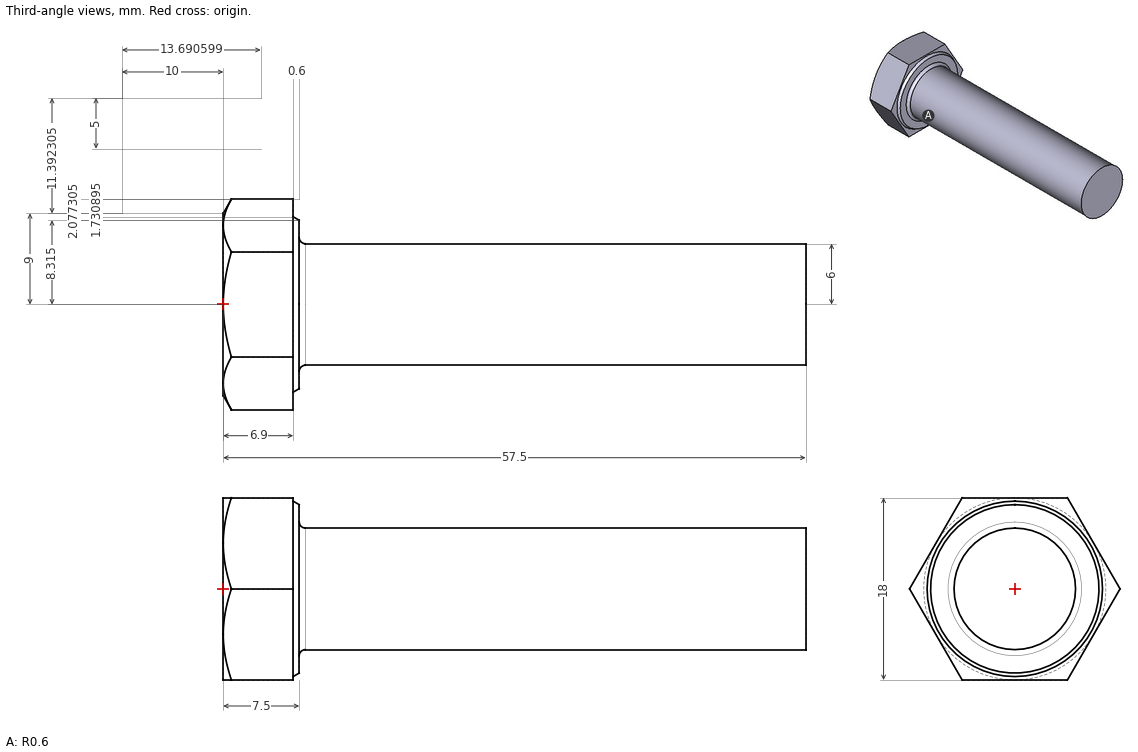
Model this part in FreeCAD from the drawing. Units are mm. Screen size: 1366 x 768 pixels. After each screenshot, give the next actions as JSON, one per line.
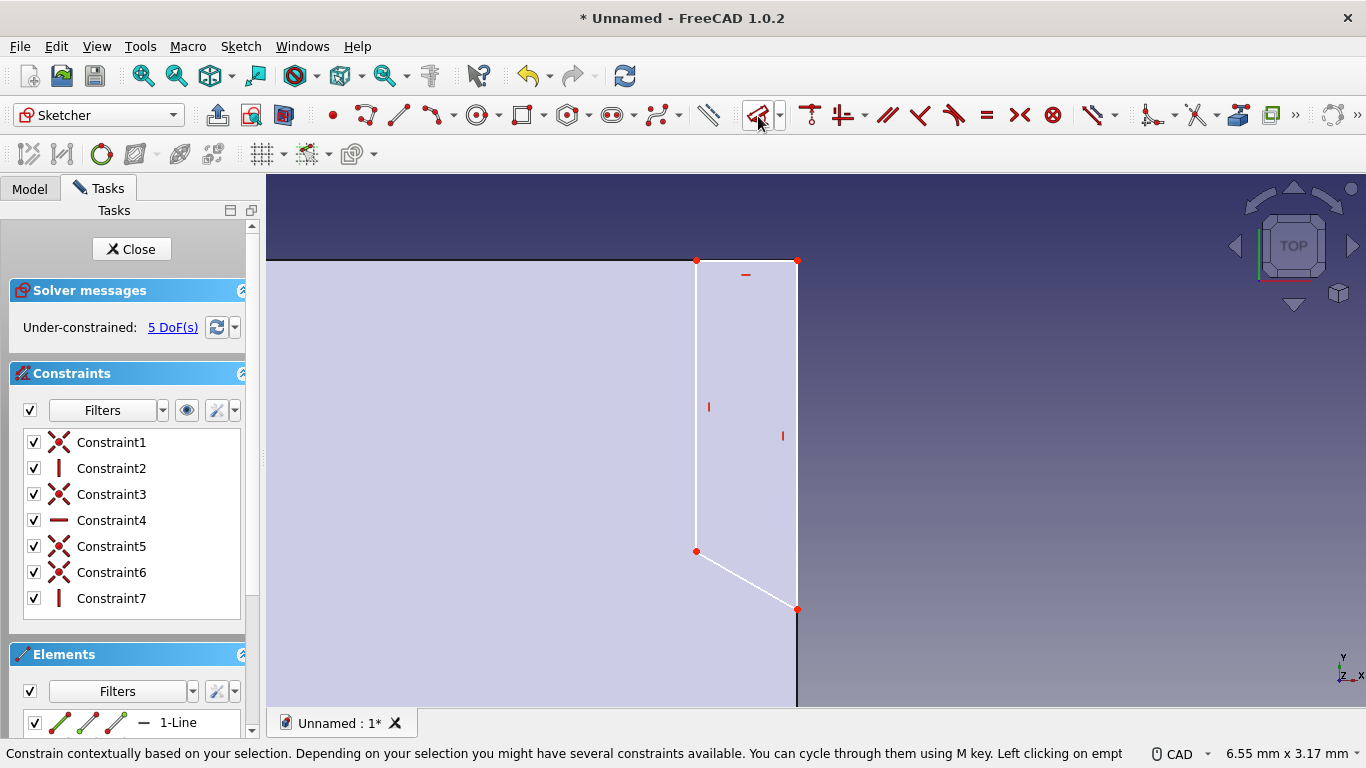
{"action": "left_click", "coordinate": [767, 261]}
{"action": "left_click", "coordinate": [746, 227]}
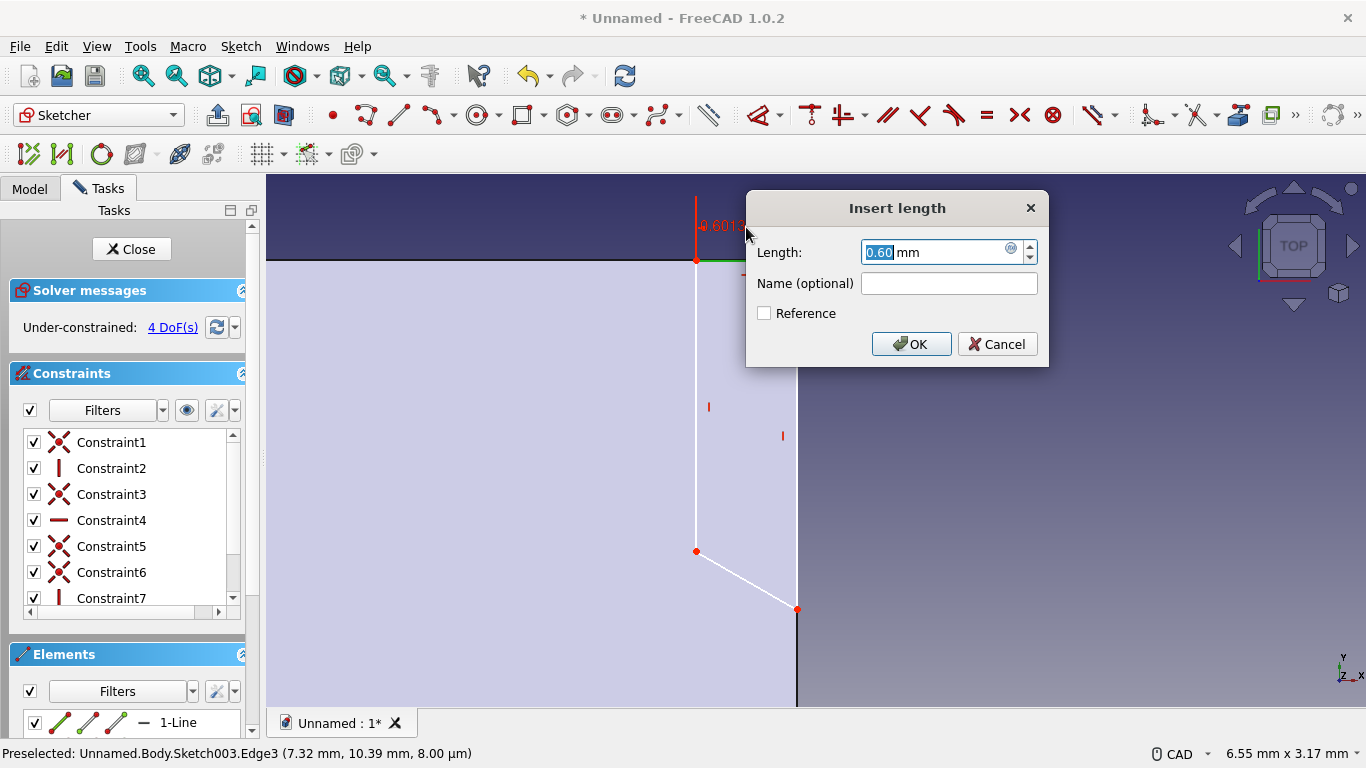
{"action": "type", "text": "0.6"}
{"action": "key", "text": "Return"}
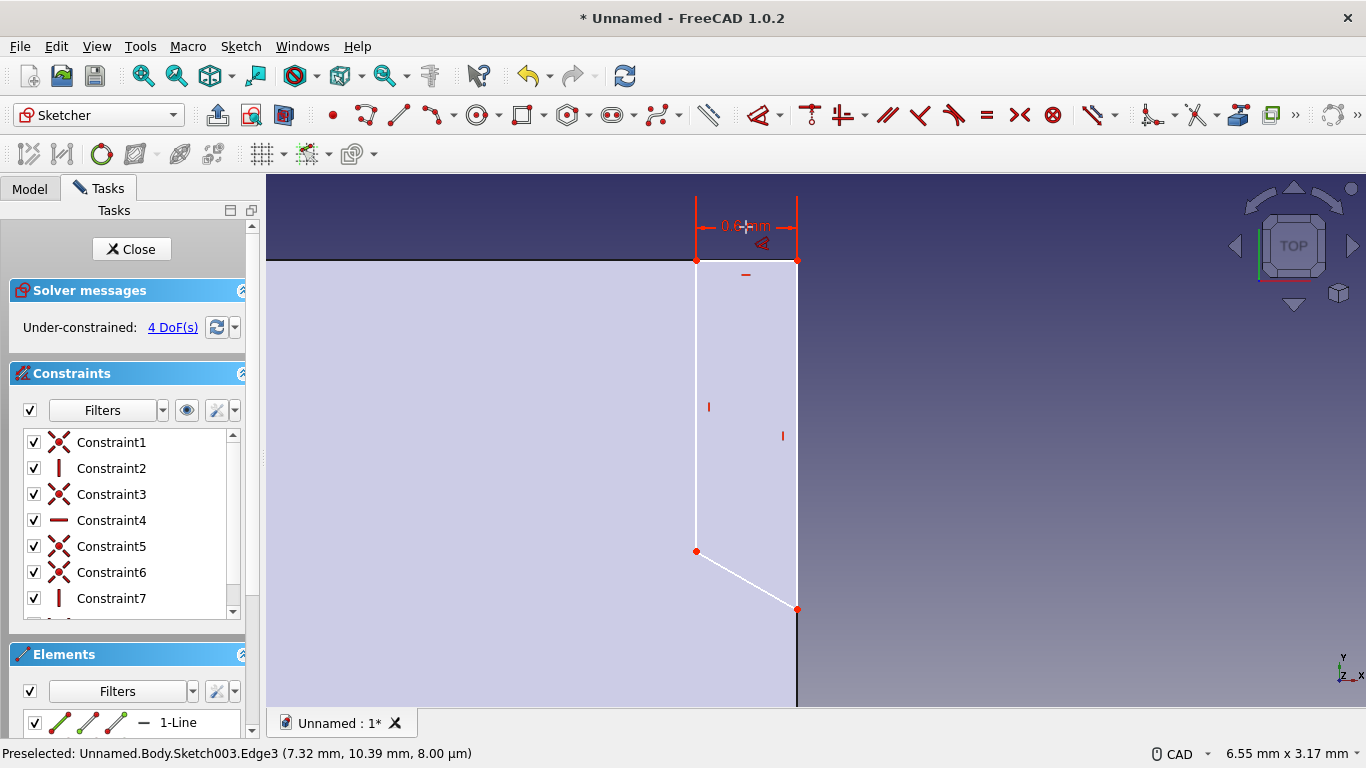
{"action": "left_click", "coordinate": [696, 552]}
{"action": "left_click", "coordinate": [495, 518]}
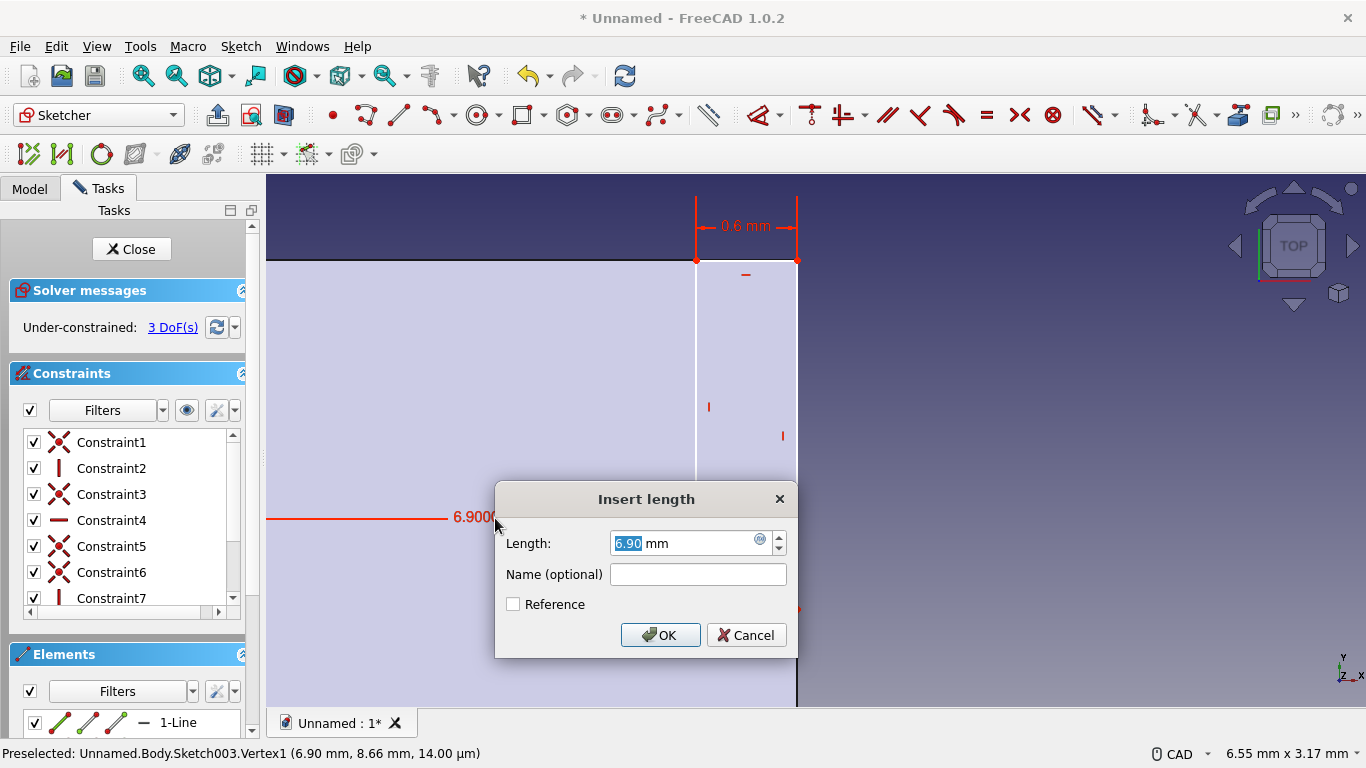
{"action": "type", "text": "6.9"}
{"action": "key", "text": "Return"}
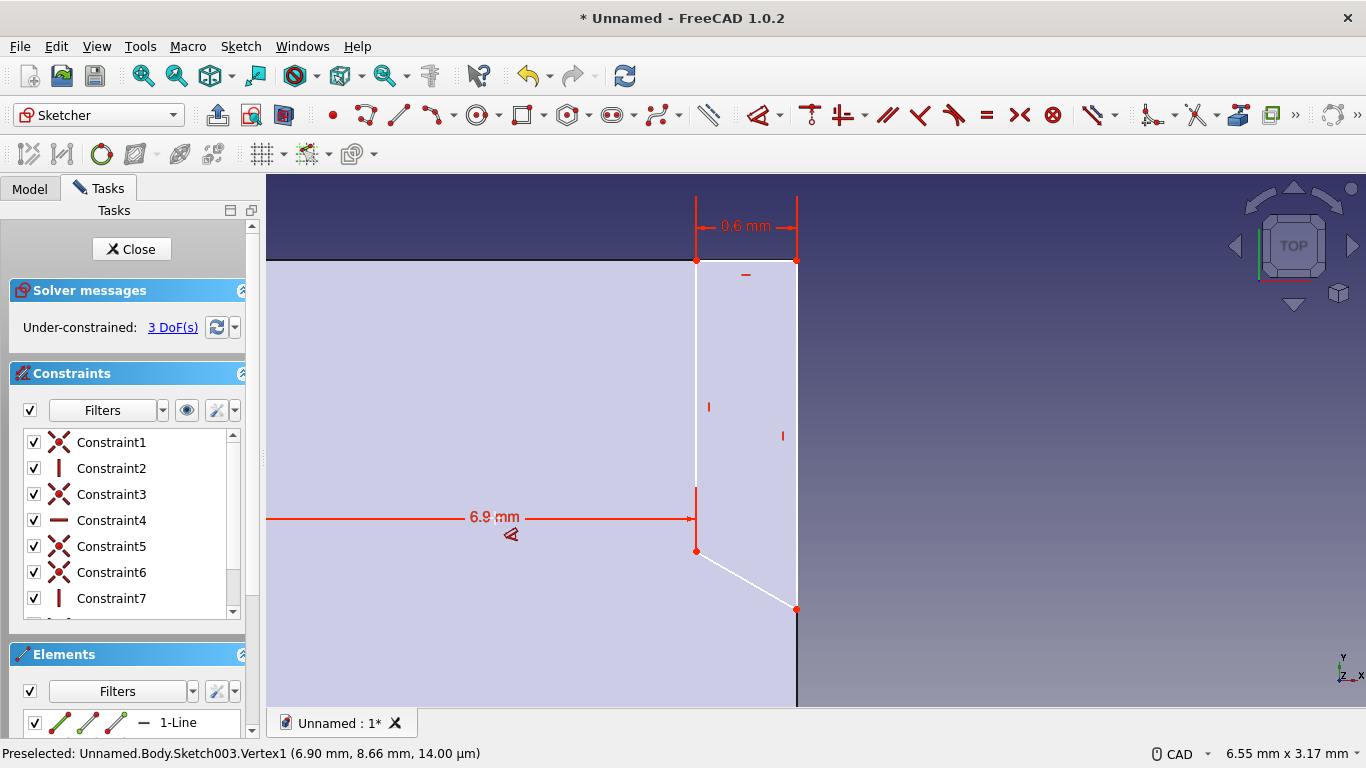
{"action": "left_click", "coordinate": [797, 610]}
{"action": "left_click", "coordinate": [831, 644]}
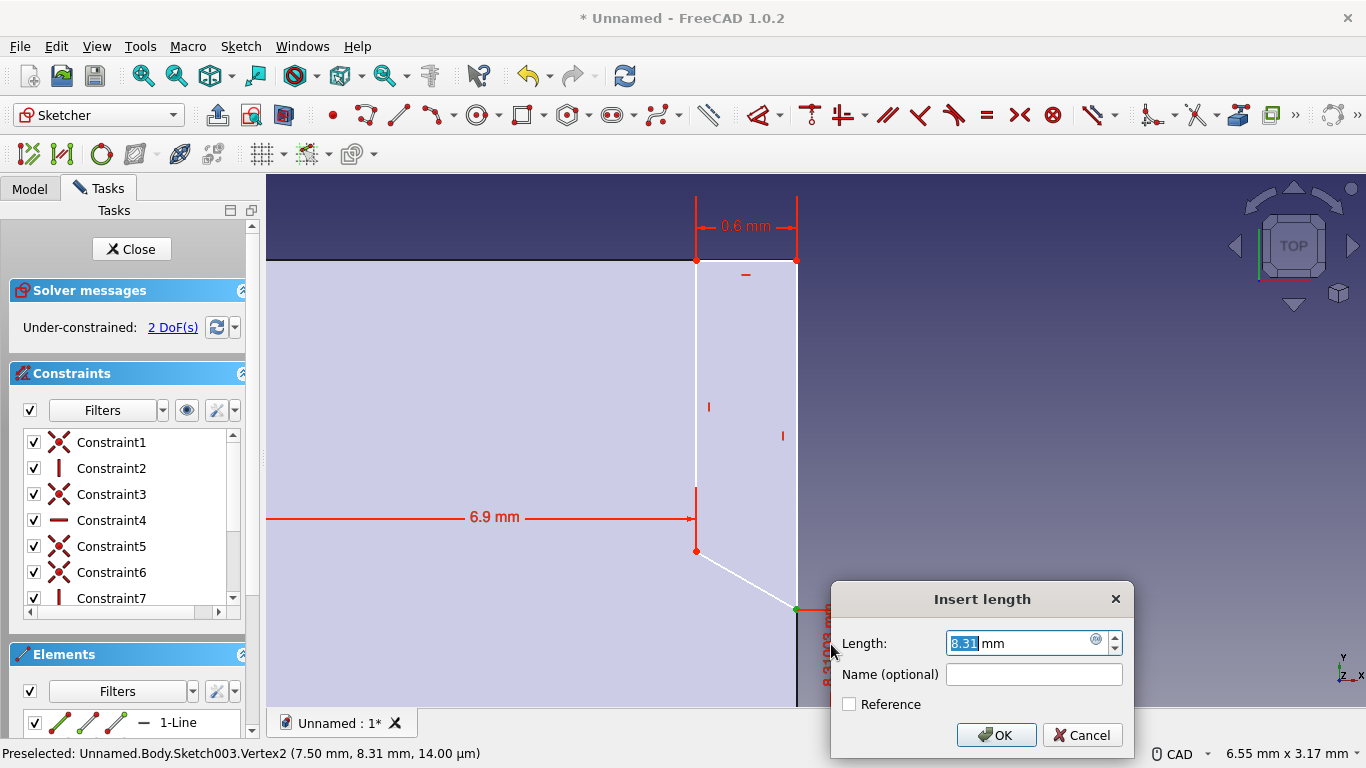
{"action": "type", "text": "8.315"}
{"action": "key", "text": "Return"}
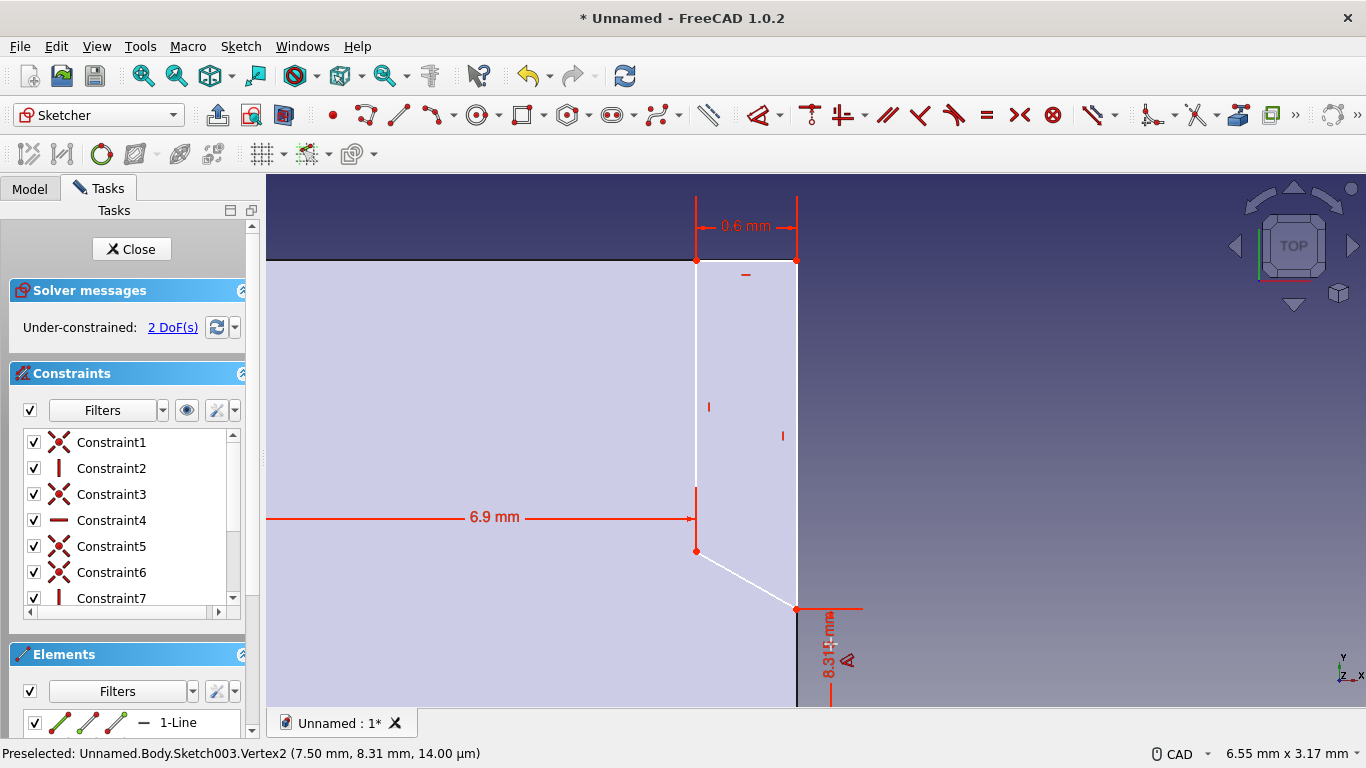
{"action": "left_click", "coordinate": [797, 505]}
{"action": "left_click", "coordinate": [831, 435]}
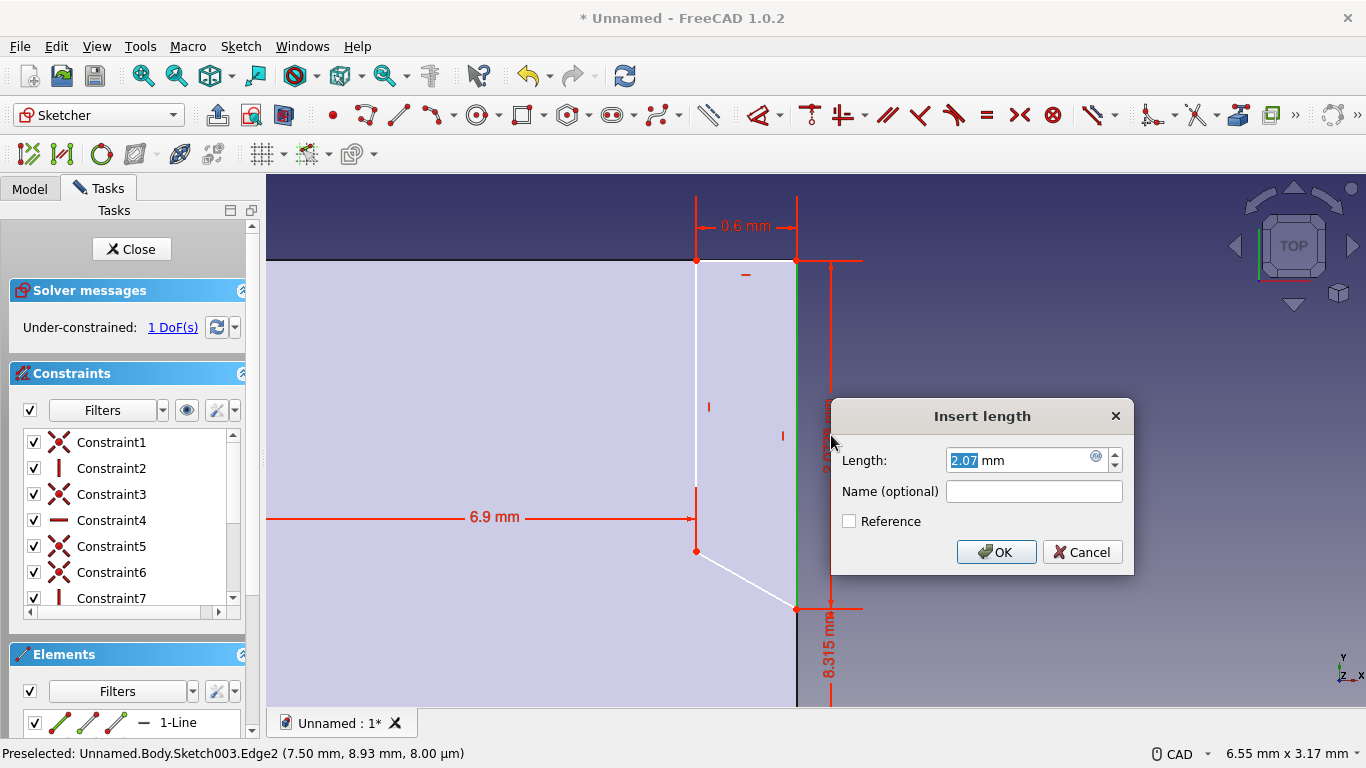
{"action": "type", "text": "2.077305"}
{"action": "key", "text": "Return"}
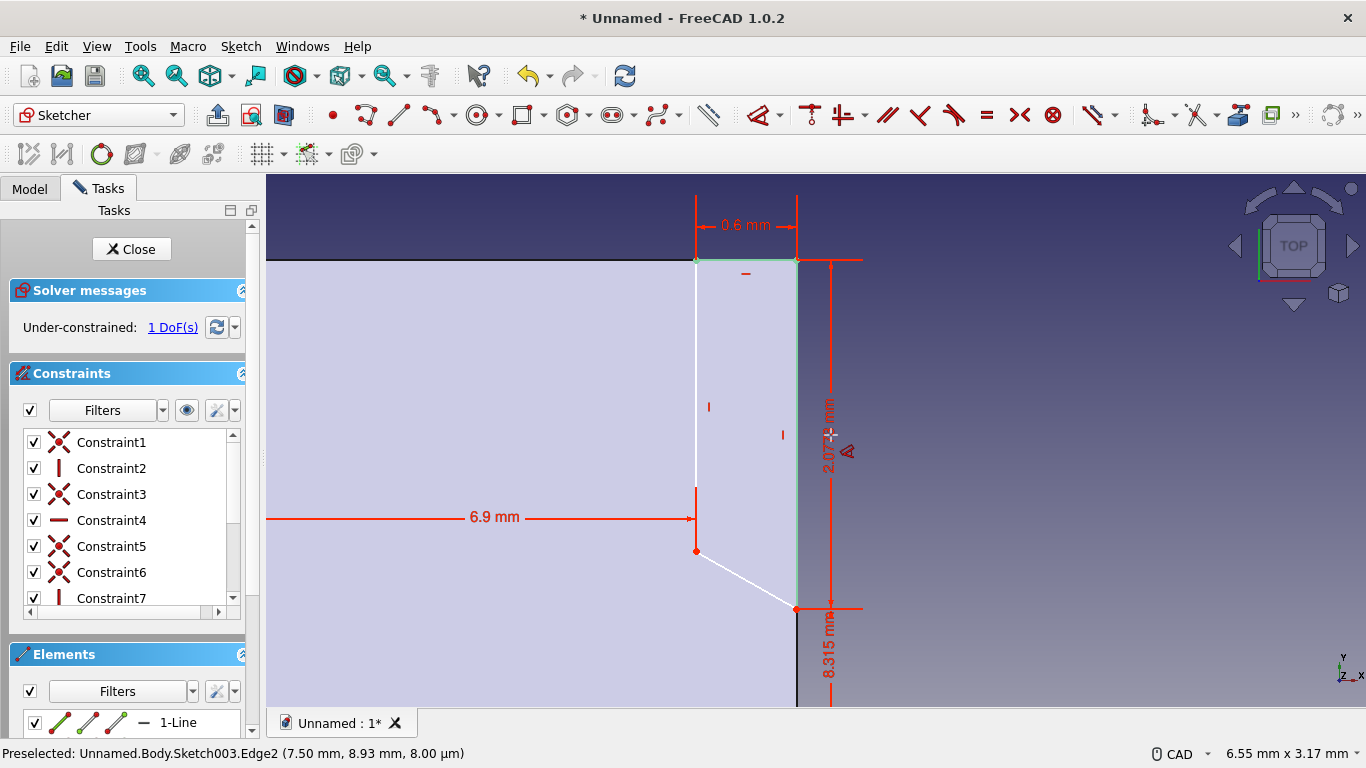
{"action": "left_click", "coordinate": [696, 348]}
{"action": "left_click", "coordinate": [662, 406]}